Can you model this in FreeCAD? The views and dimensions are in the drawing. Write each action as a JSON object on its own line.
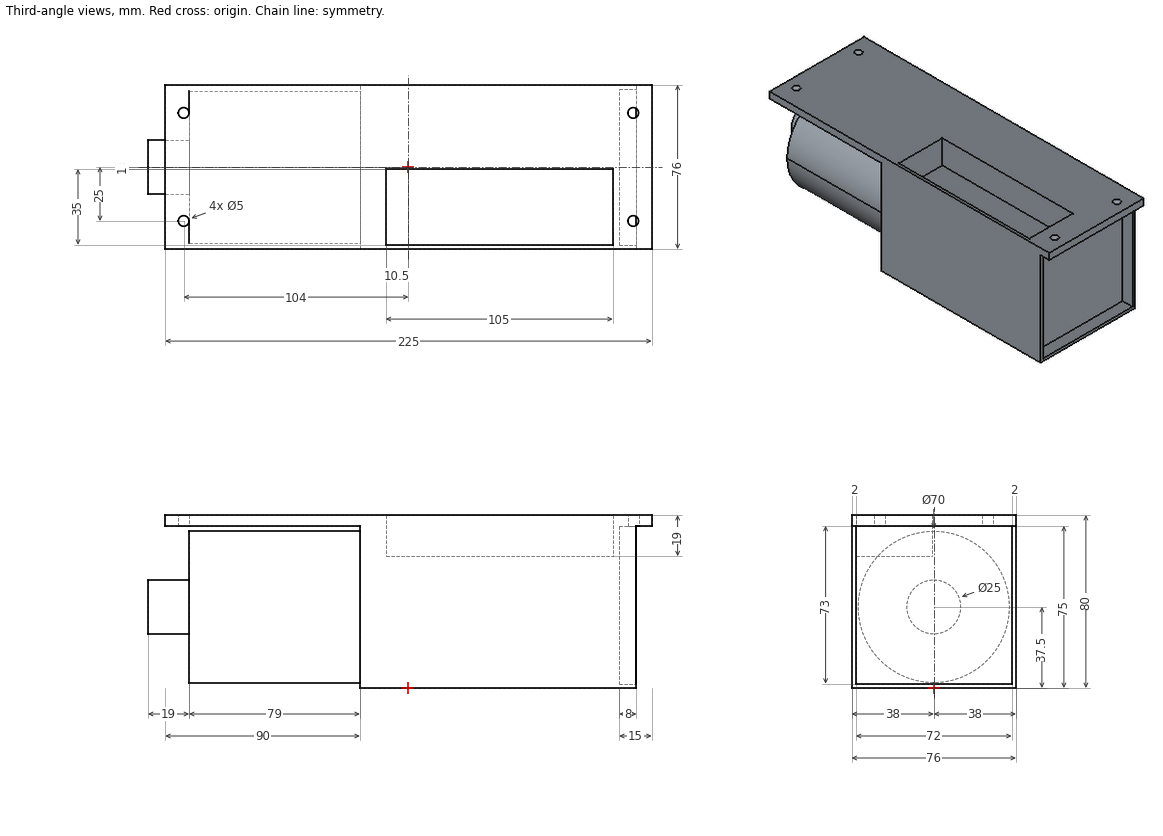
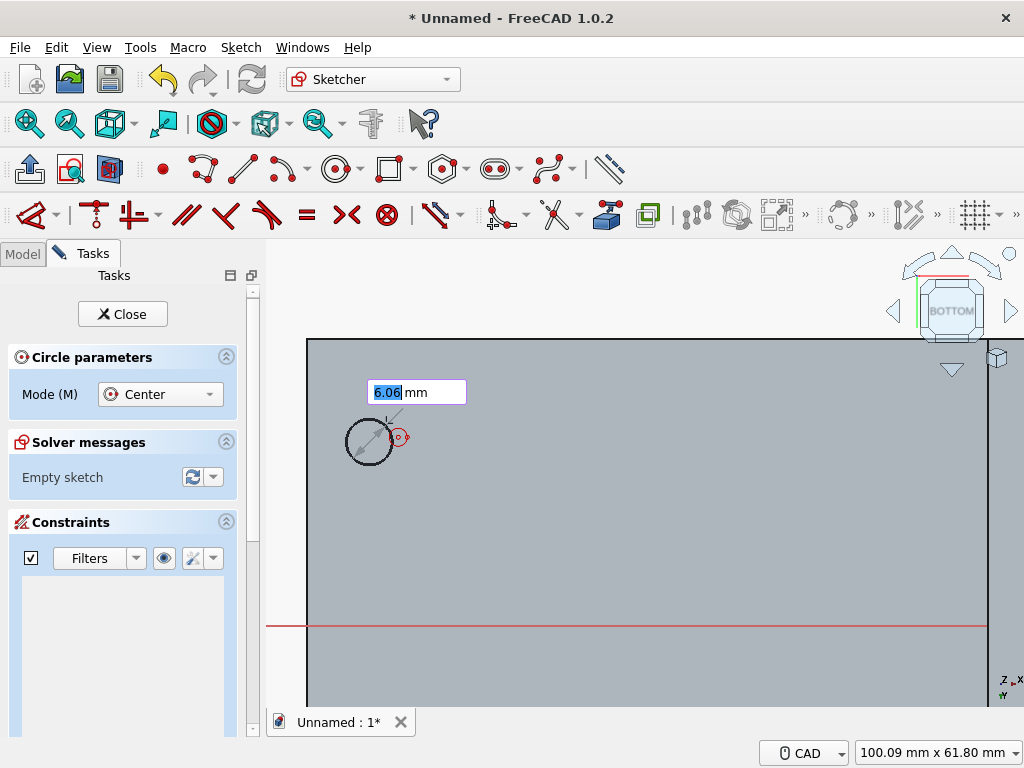
{"action": "left_click", "coordinate": [384, 424]}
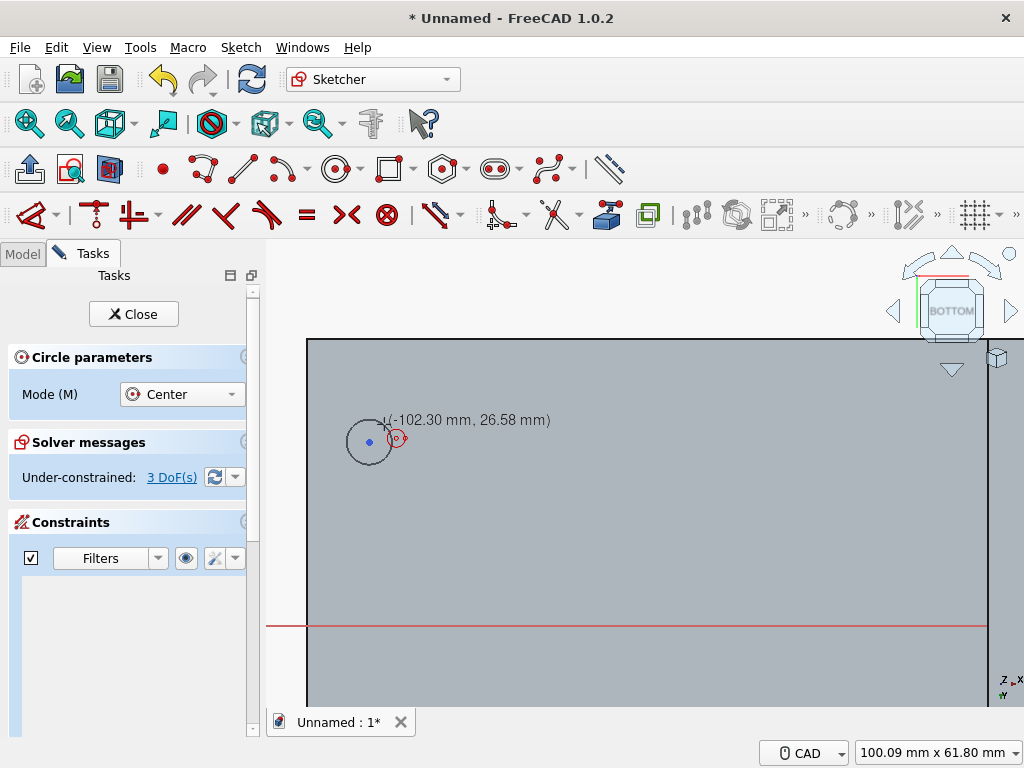
{"action": "scroll", "coordinate": [386, 423], "scroll_direction": "down", "scroll_amount": 7}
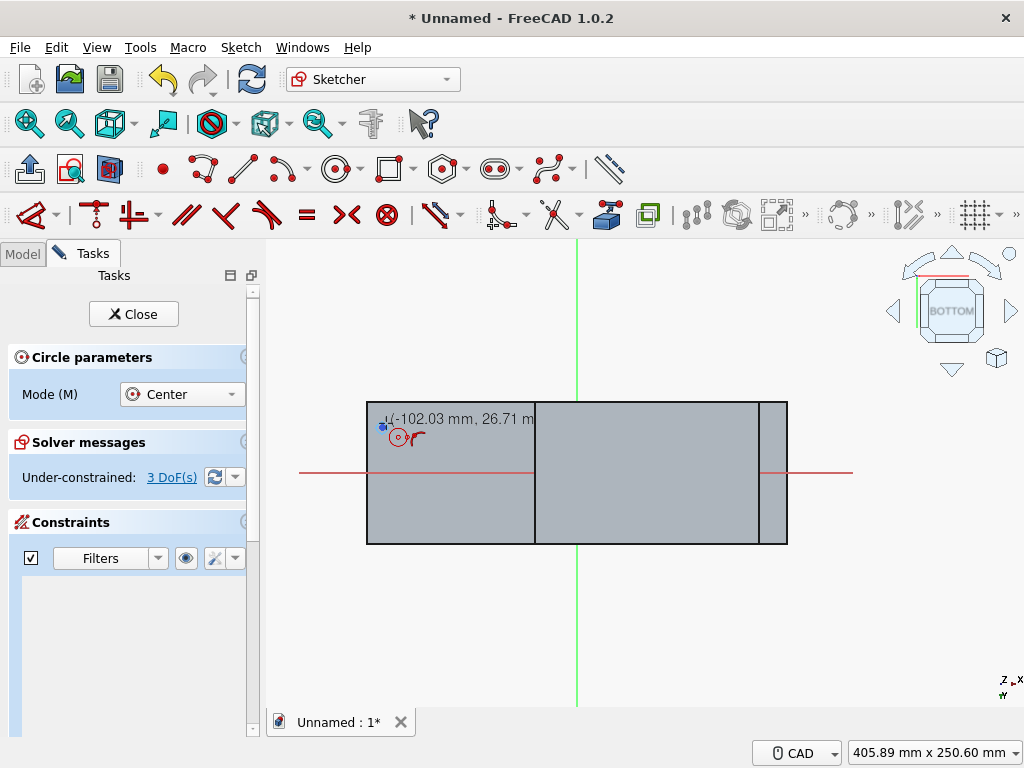
{"action": "scroll", "coordinate": [382, 520], "scroll_direction": "up", "scroll_amount": 8}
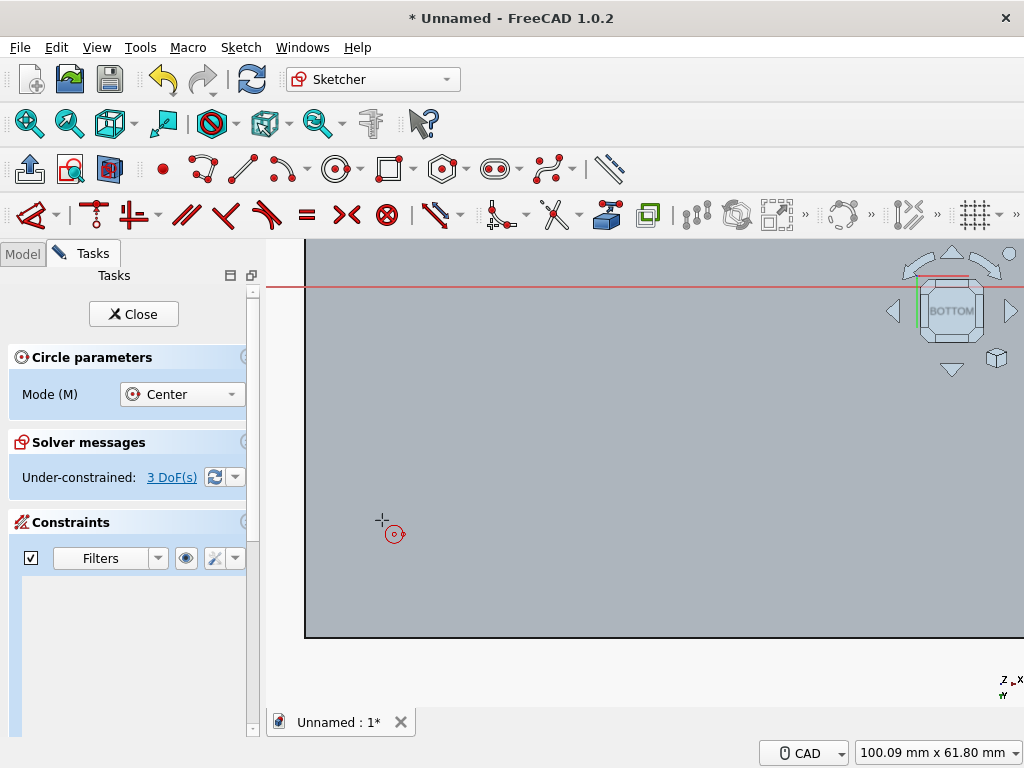
{"action": "scroll", "coordinate": [382, 520], "scroll_direction": "down", "scroll_amount": 8}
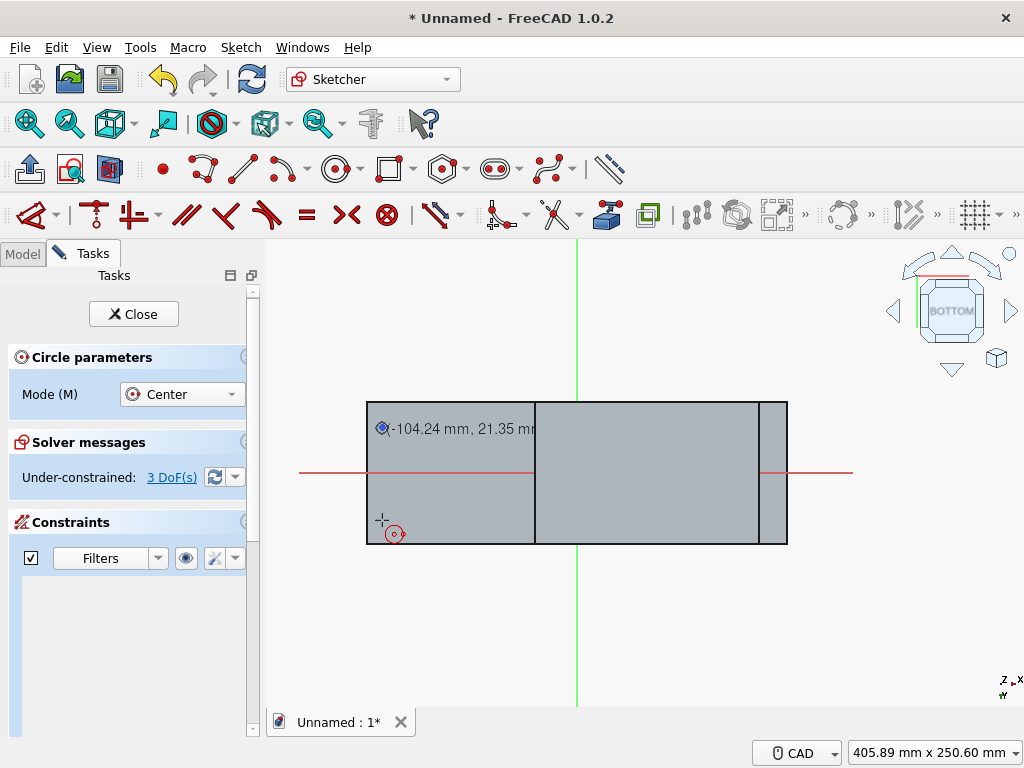
{"action": "left_click", "coordinate": [382, 520]}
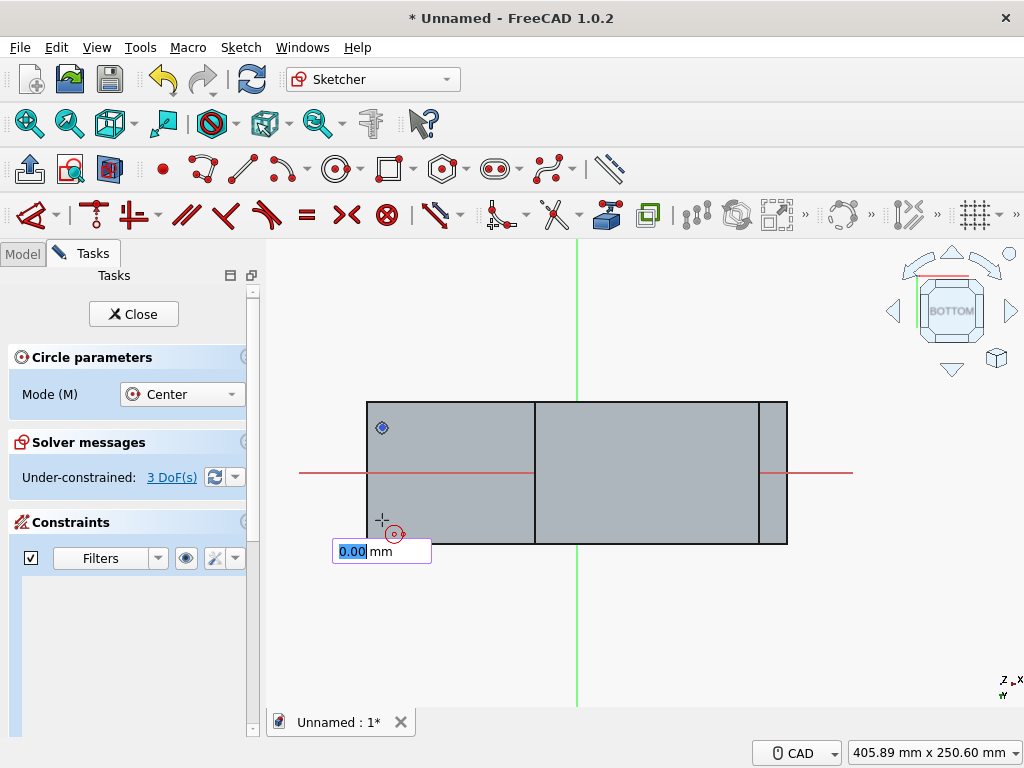
{"action": "scroll", "coordinate": [386, 517], "scroll_direction": "up", "scroll_amount": 7}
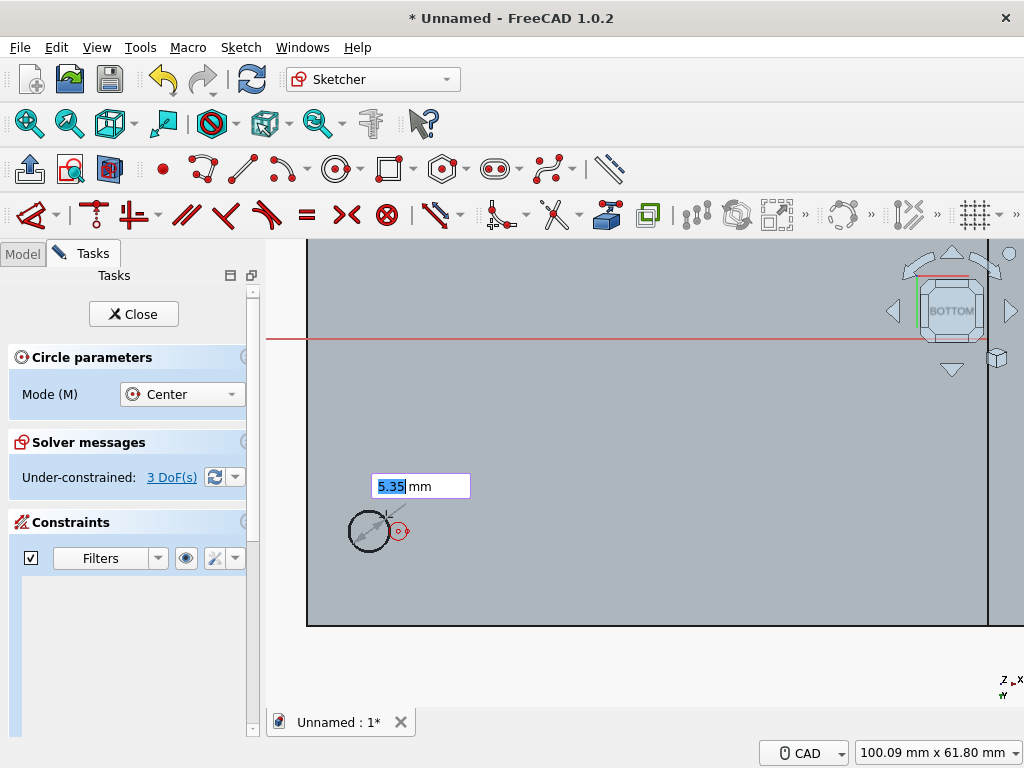
{"action": "left_click", "coordinate": [384, 514]}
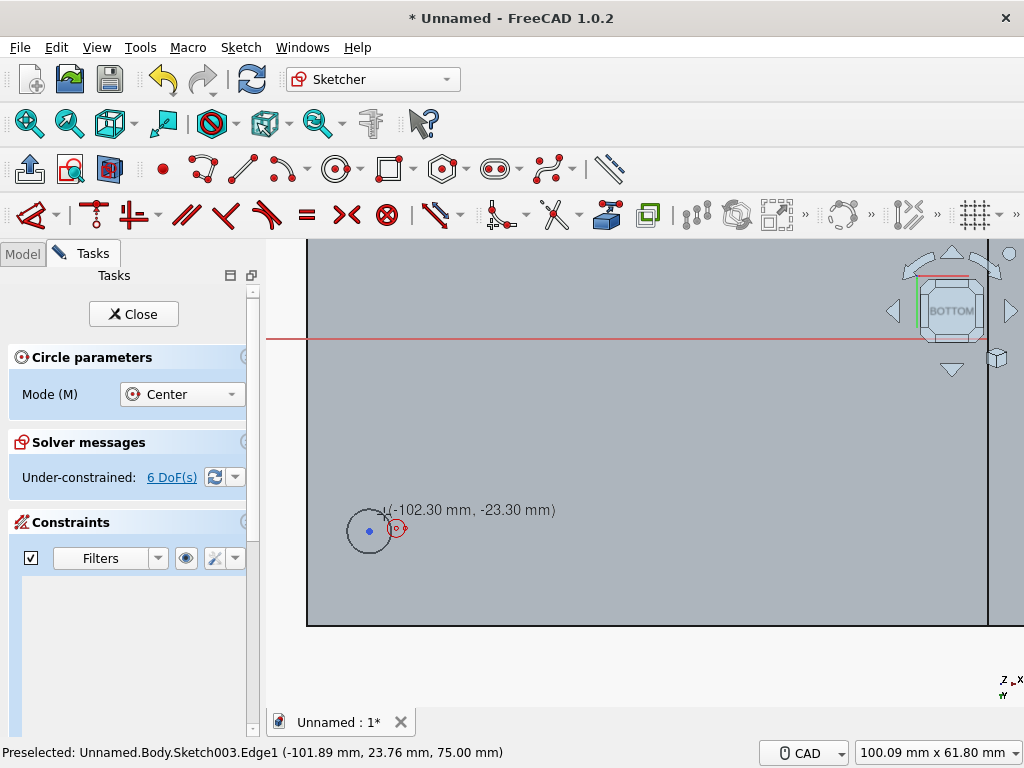
{"action": "scroll", "coordinate": [386, 517], "scroll_direction": "down", "scroll_amount": 7}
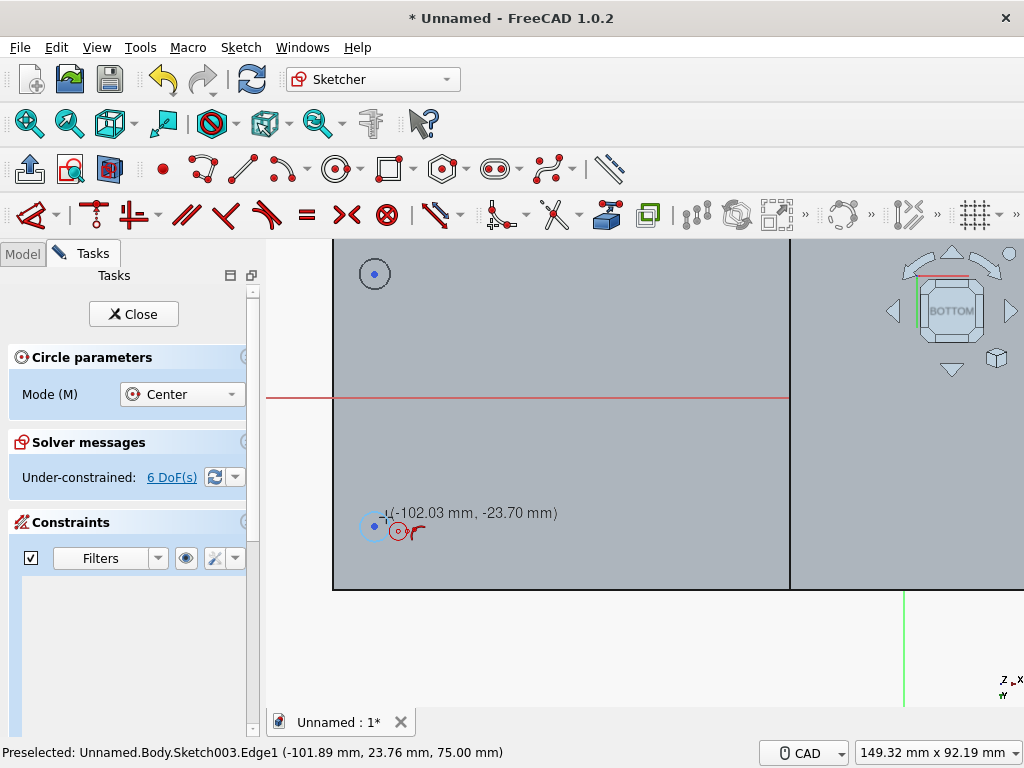
{"action": "scroll", "coordinate": [771, 427], "scroll_direction": "up", "scroll_amount": 8}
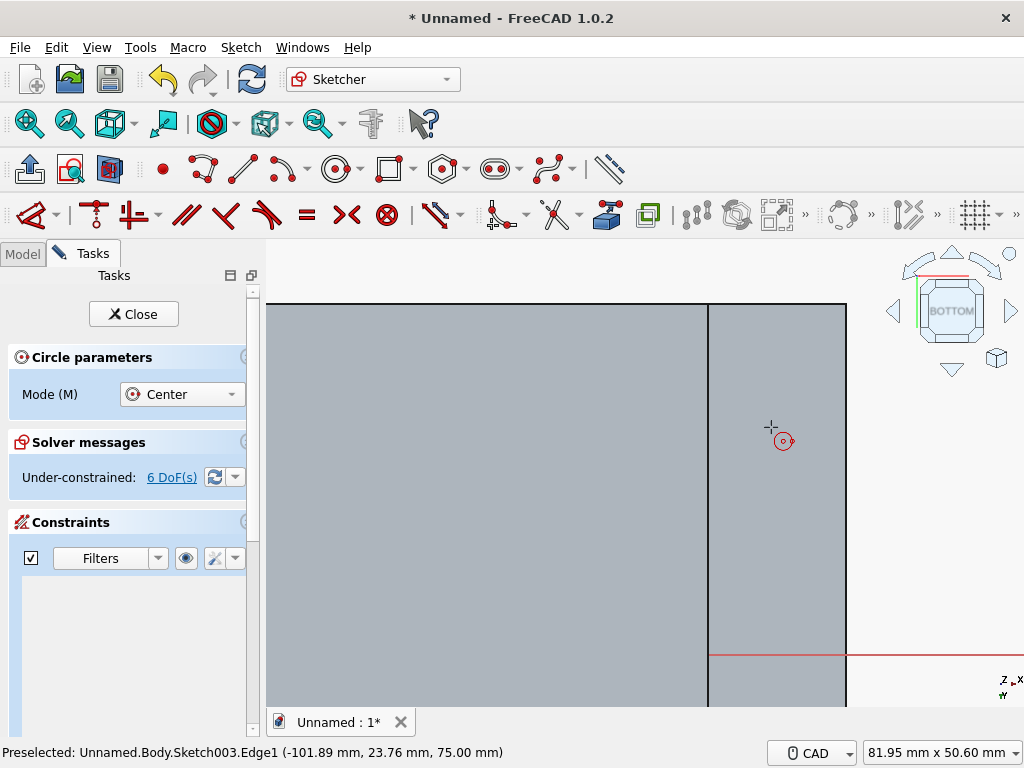
{"action": "scroll", "coordinate": [771, 427], "scroll_direction": "down", "scroll_amount": 8}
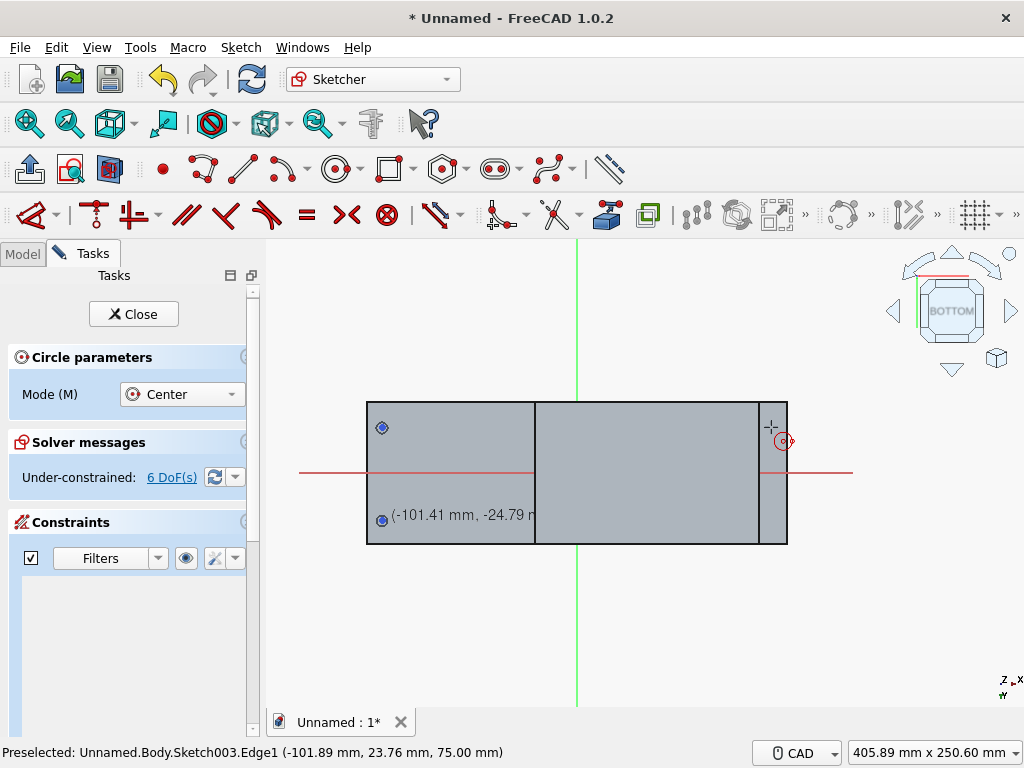
{"action": "left_click", "coordinate": [771, 427]}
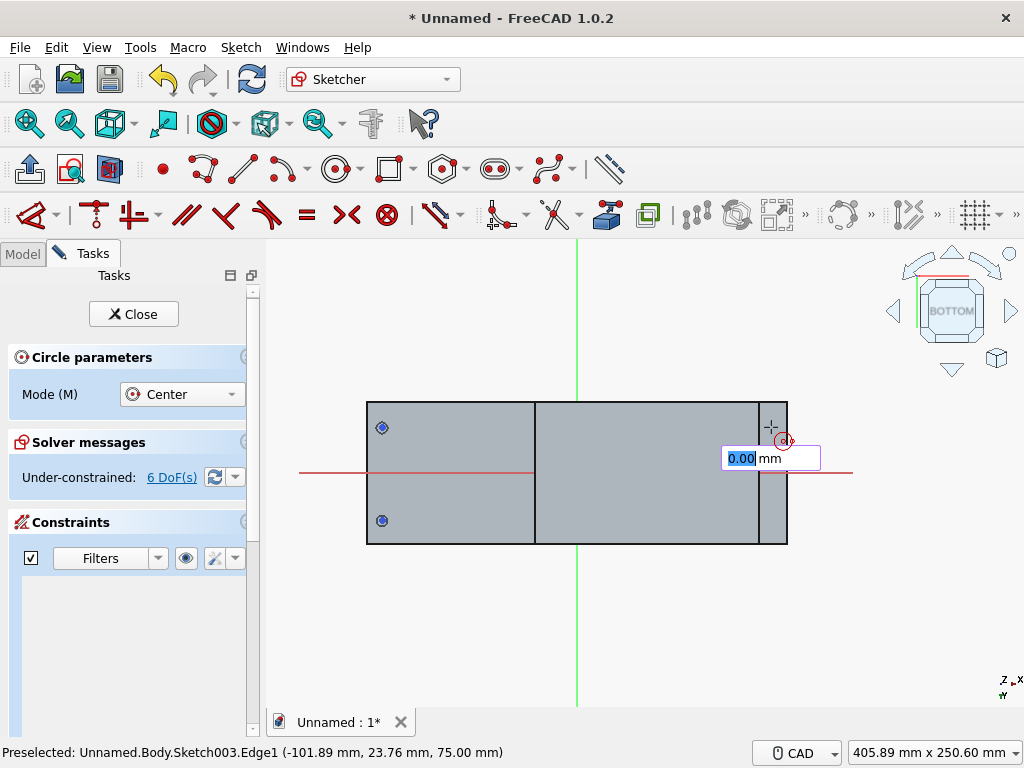
{"action": "scroll", "coordinate": [774, 423], "scroll_direction": "up", "scroll_amount": 7}